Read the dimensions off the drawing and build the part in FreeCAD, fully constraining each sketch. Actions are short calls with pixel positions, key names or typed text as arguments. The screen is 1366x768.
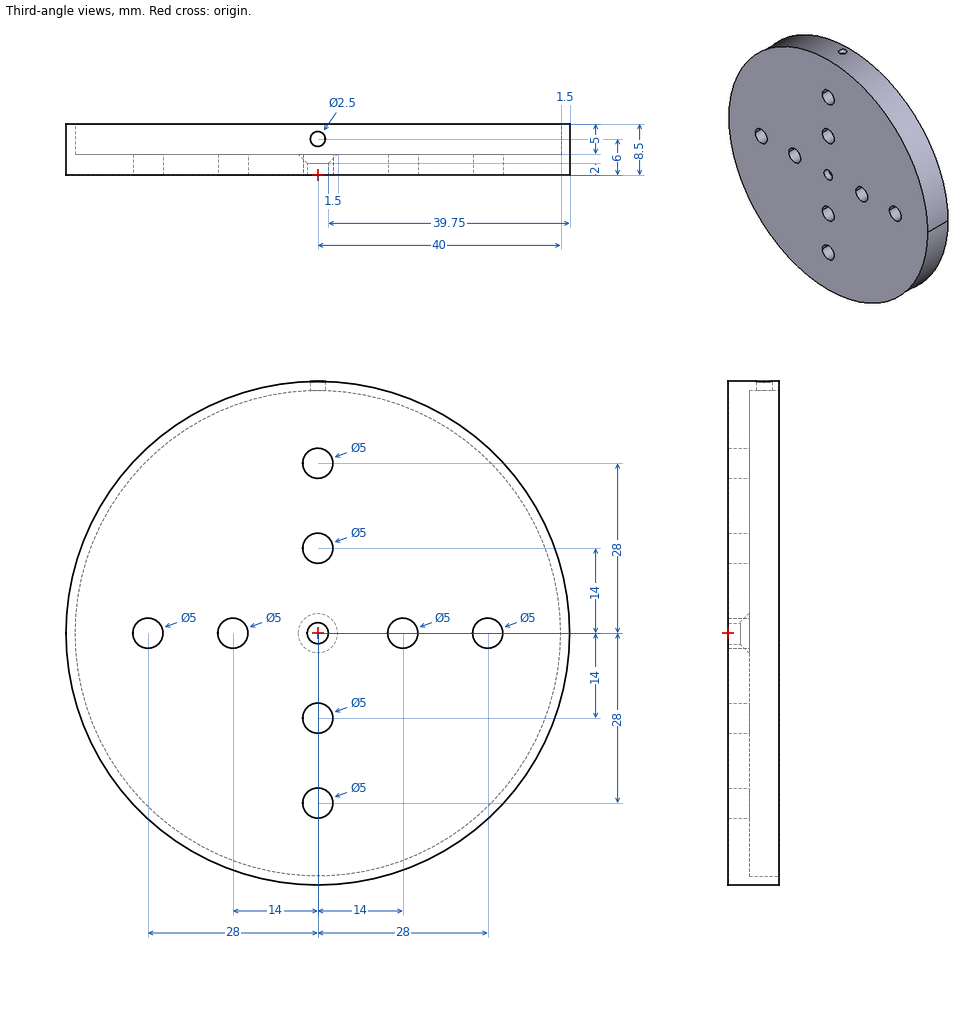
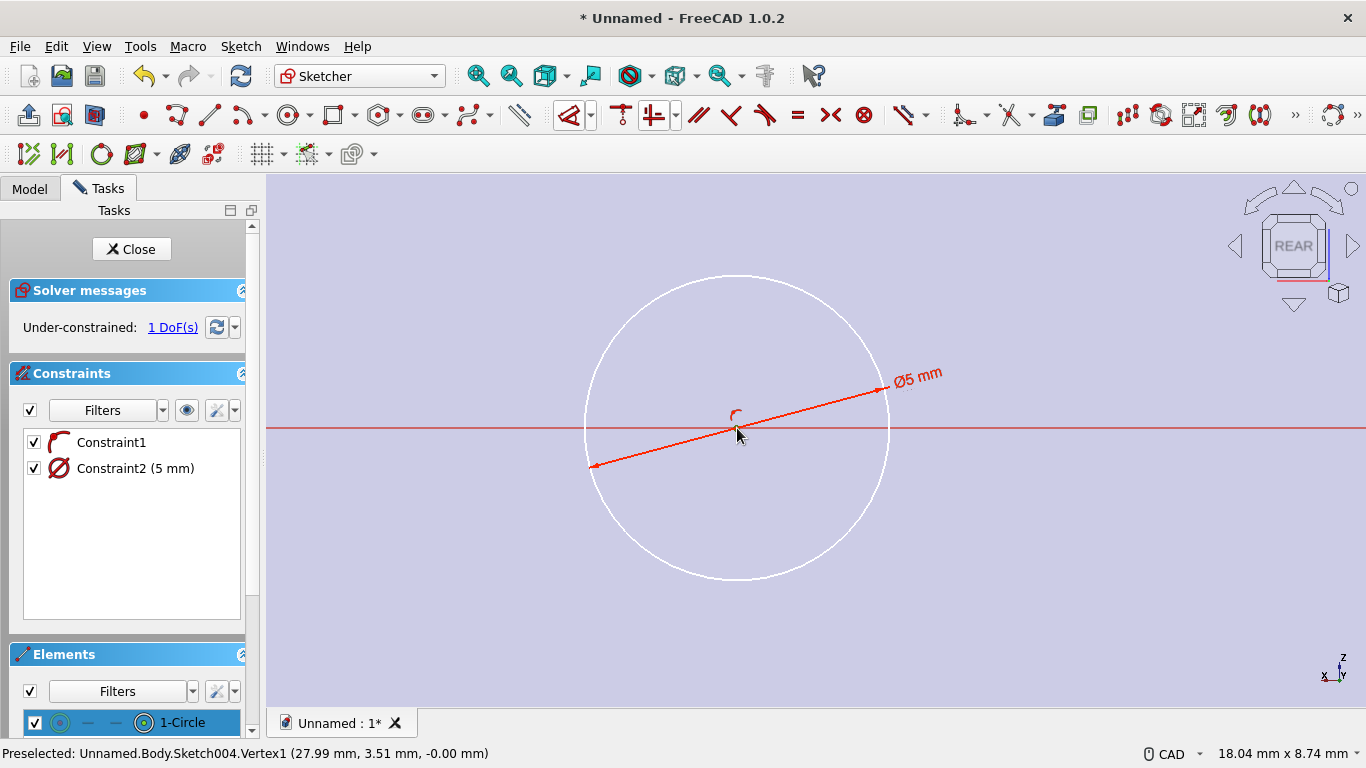
click(590, 116)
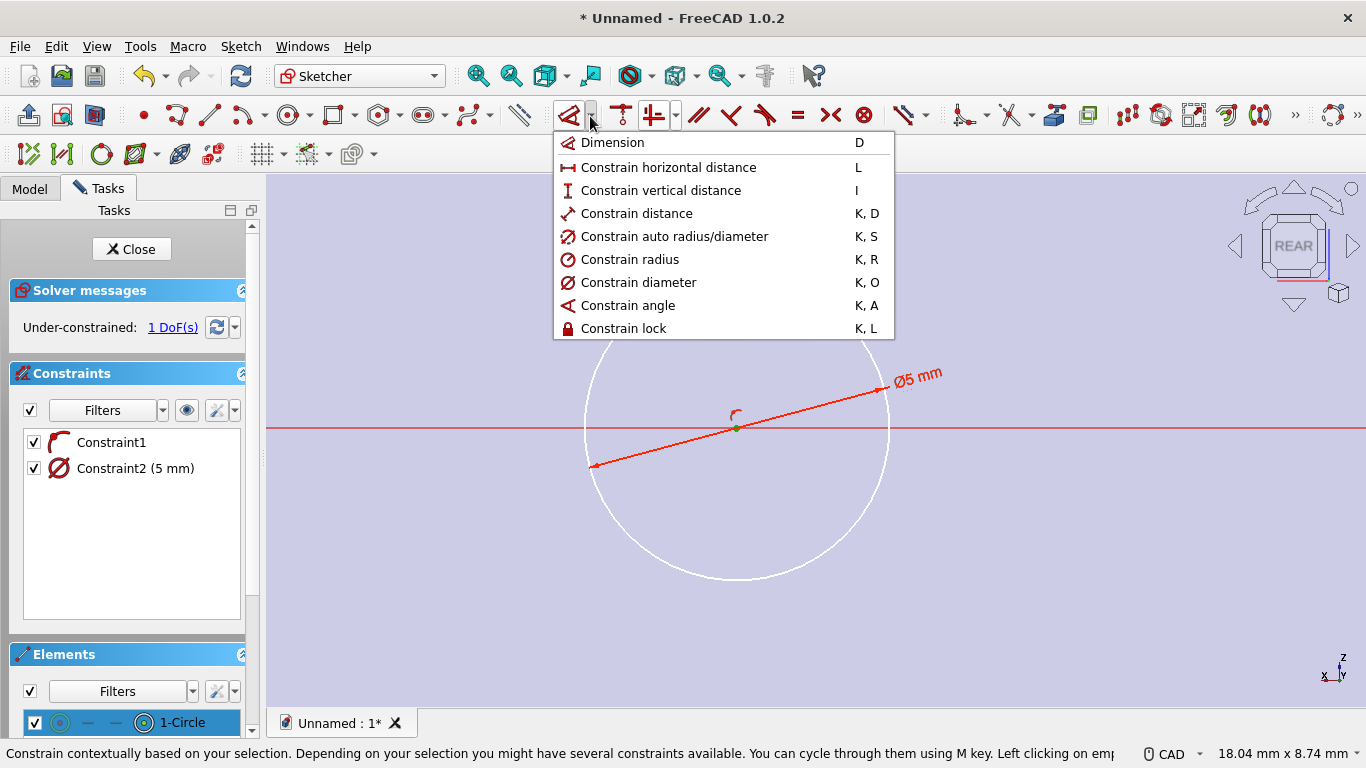
click(724, 168)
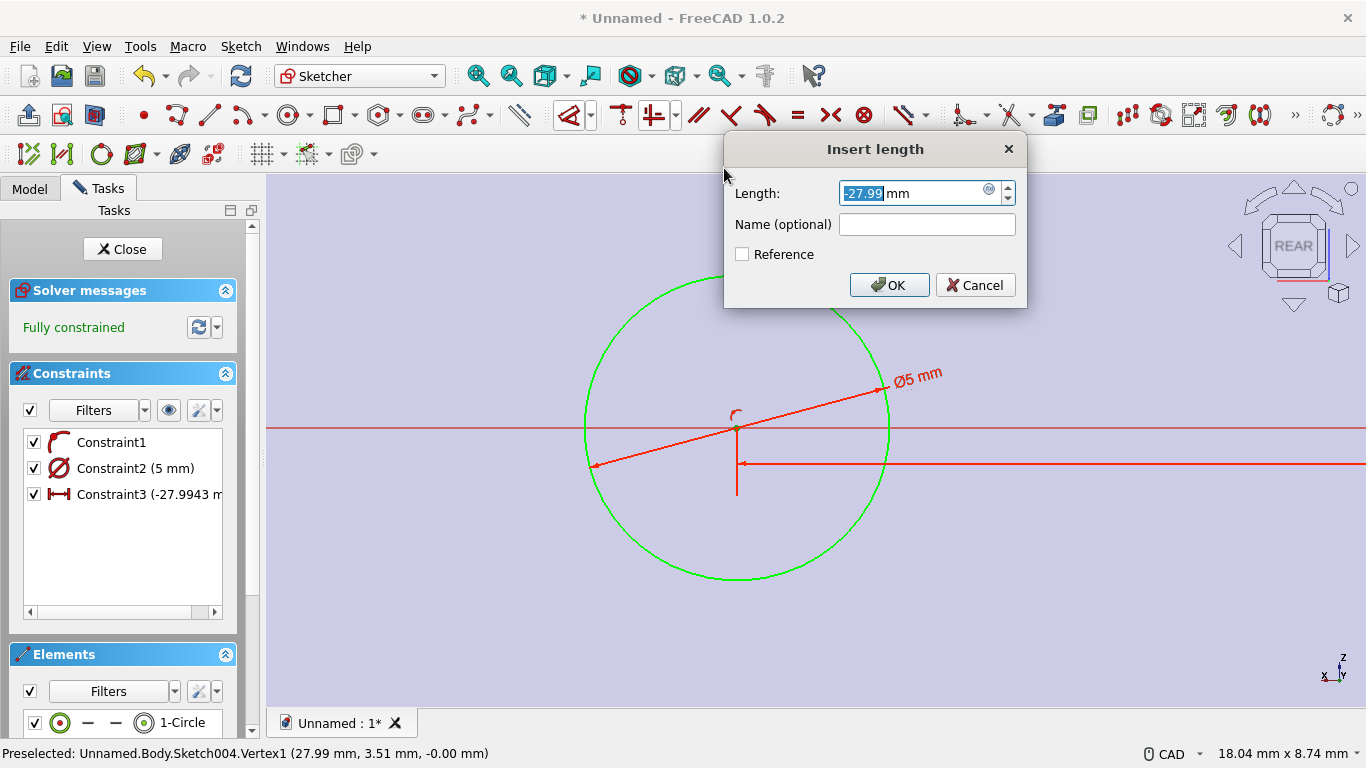
text(-28)
key(Return)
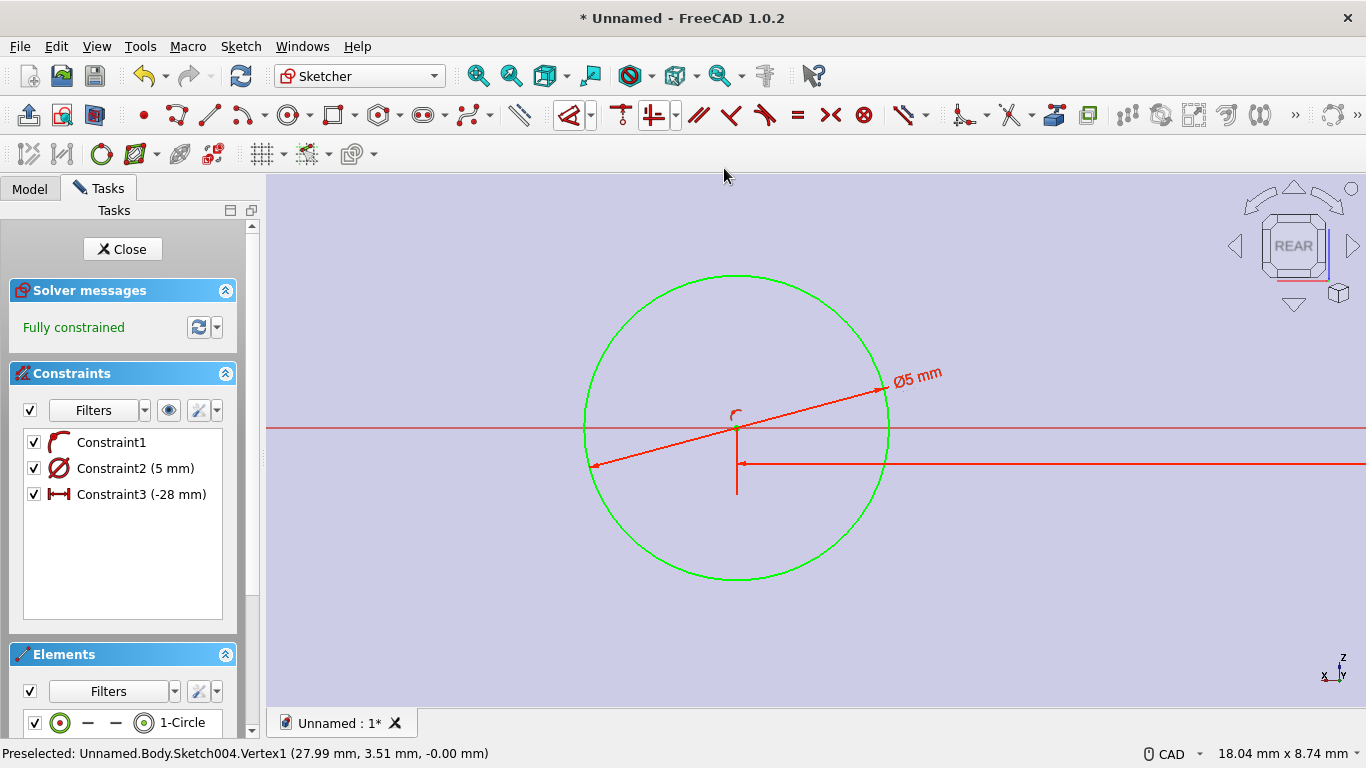
click(123, 249)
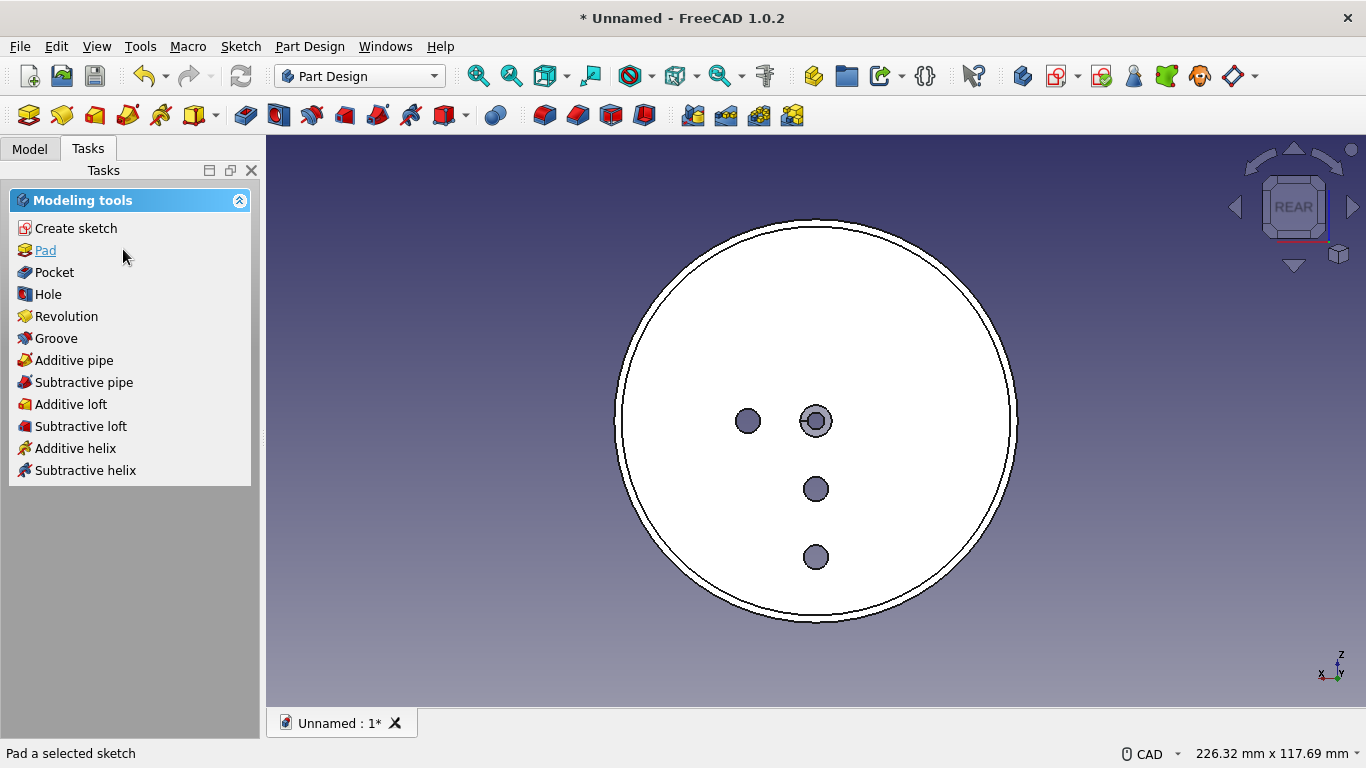
click(246, 116)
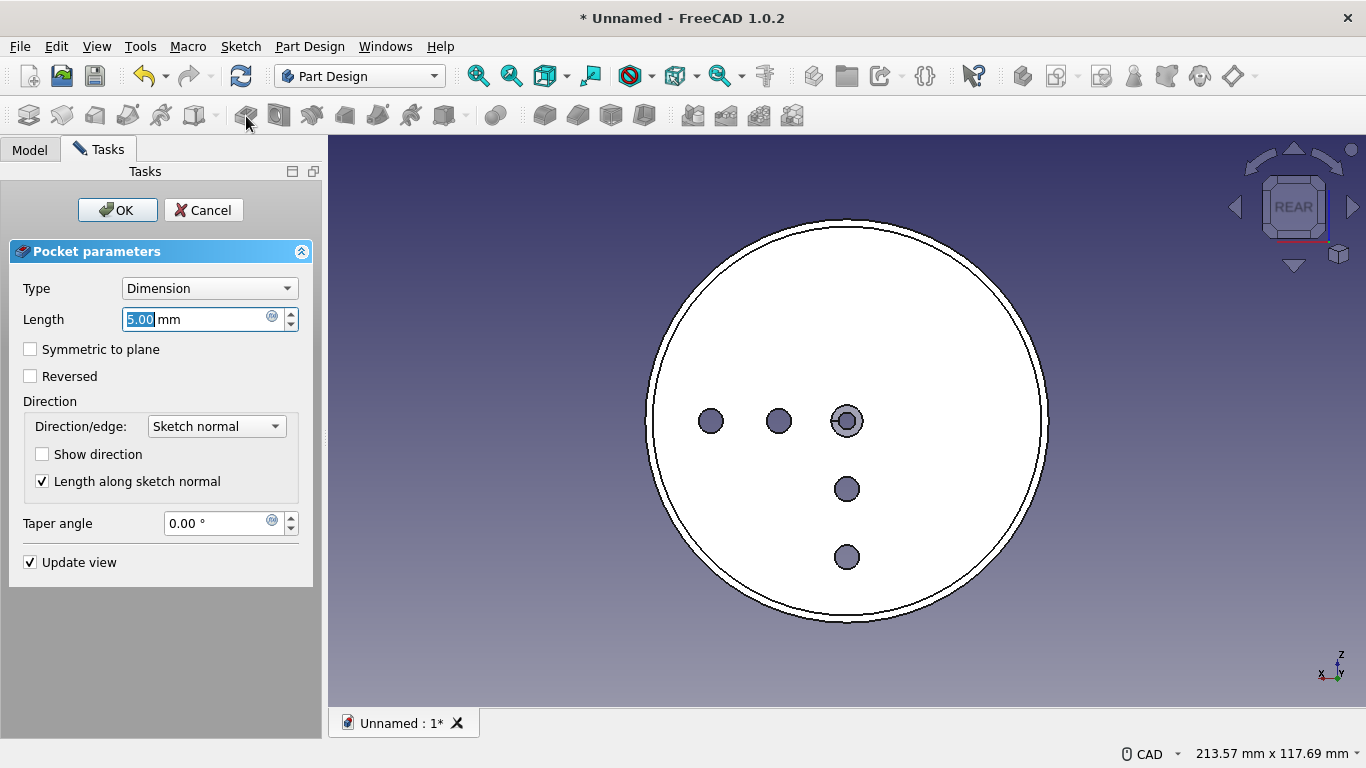
click(210, 288)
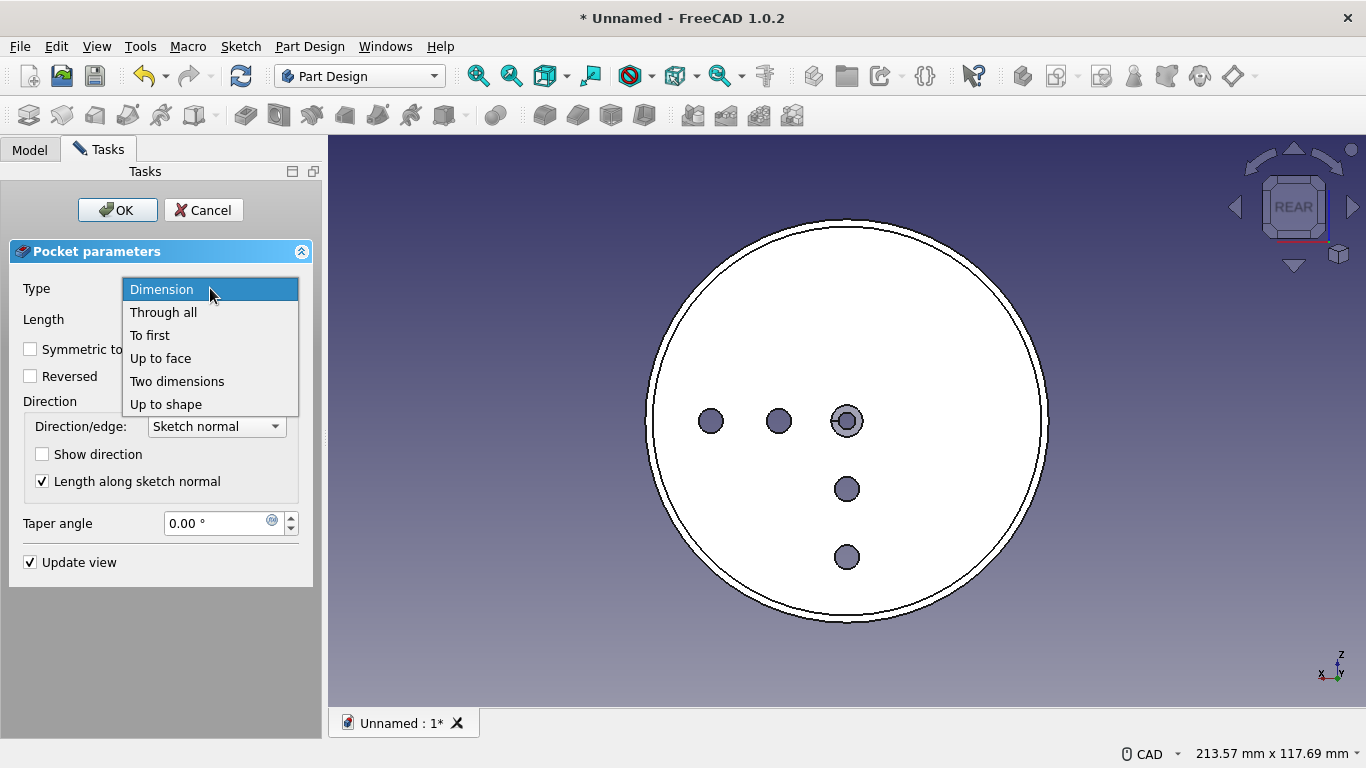
click(208, 336)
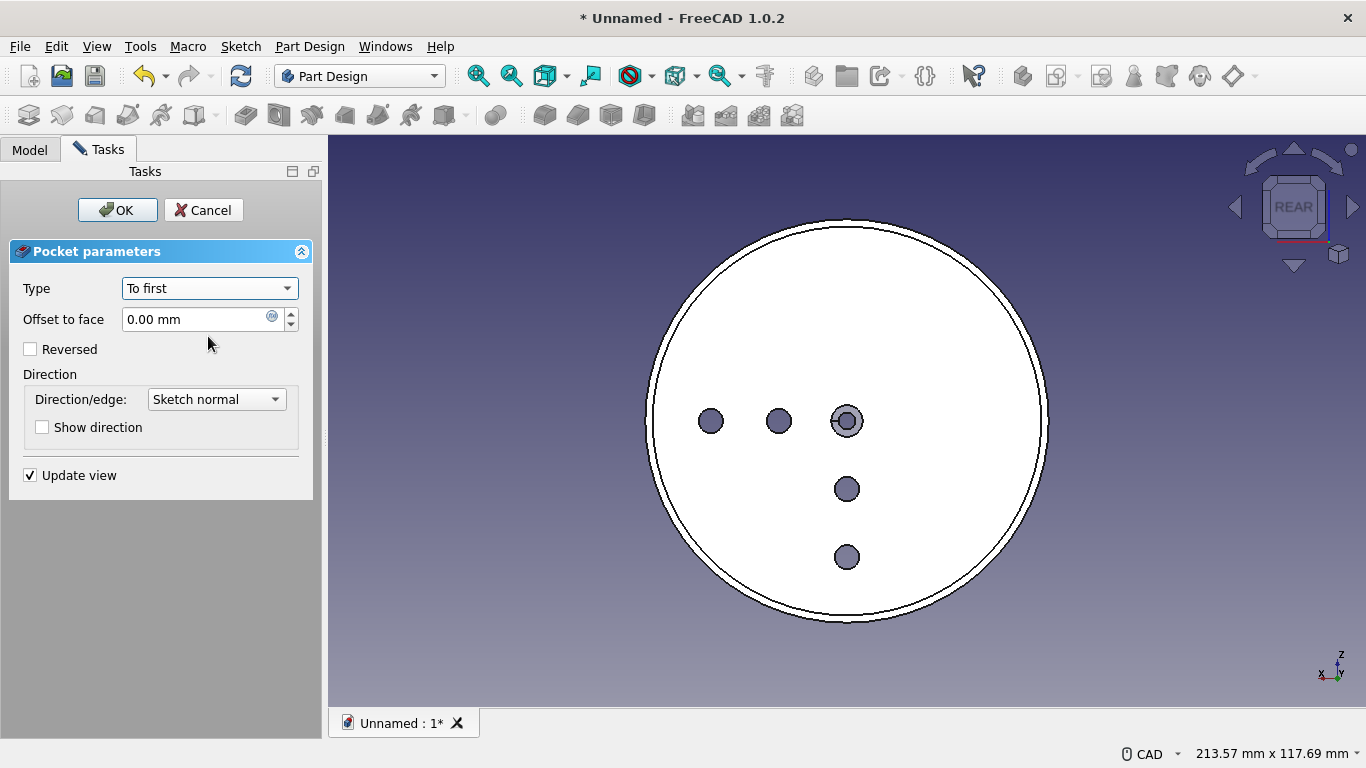
click(118, 210)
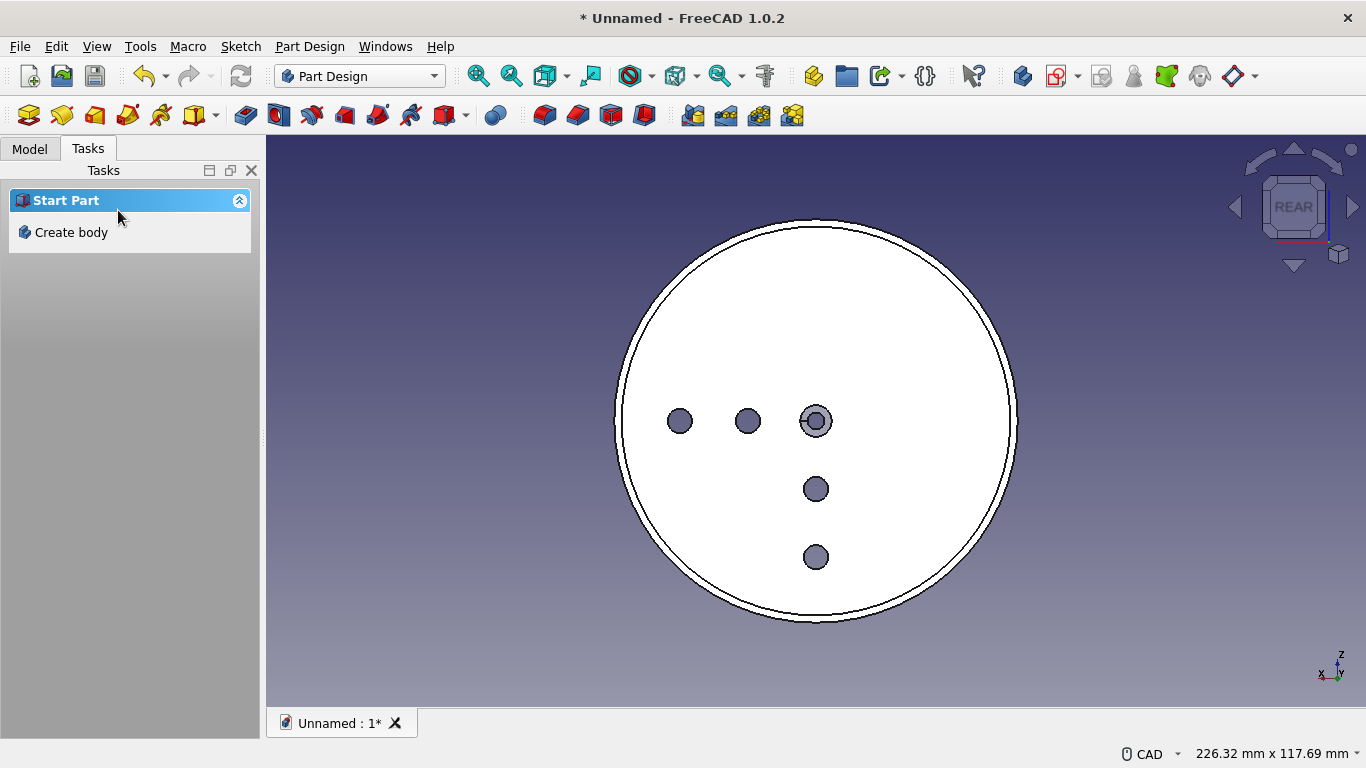
click(816, 309)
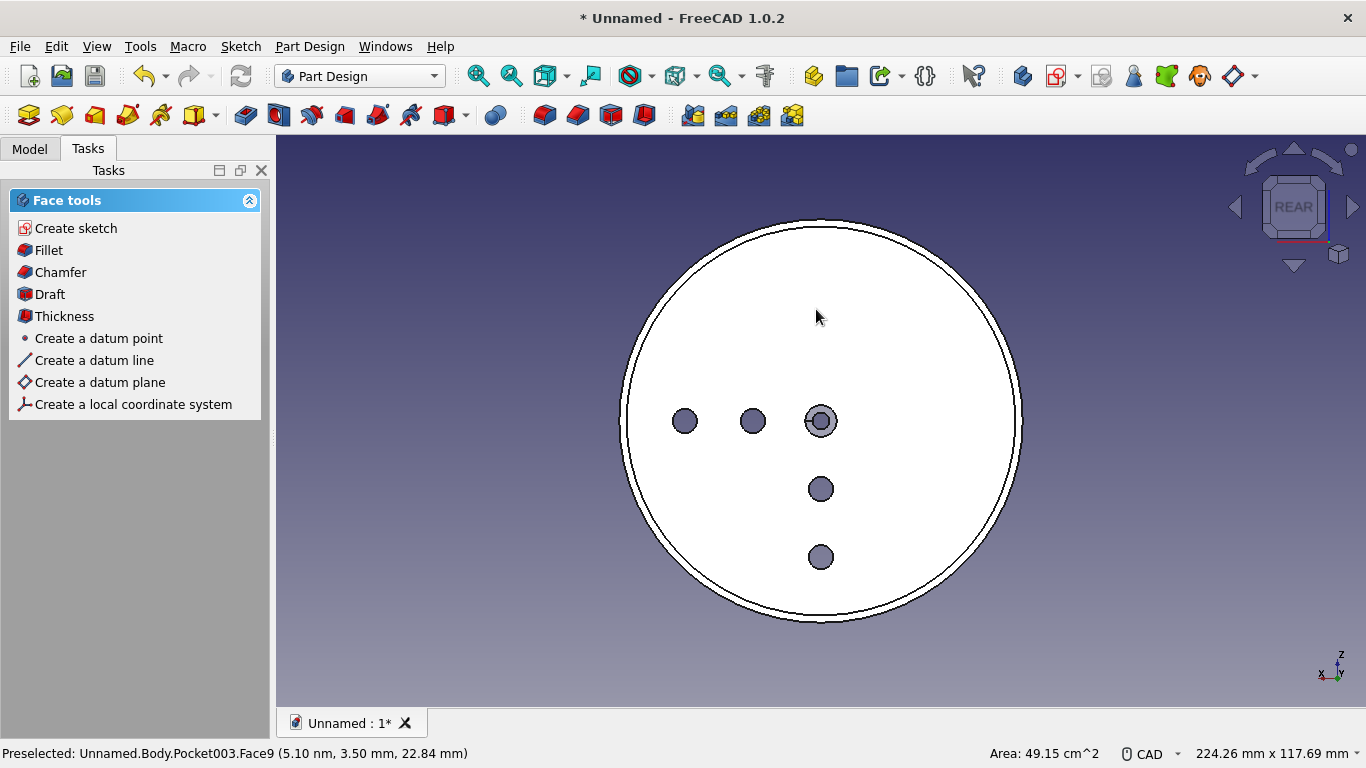
click(1056, 76)